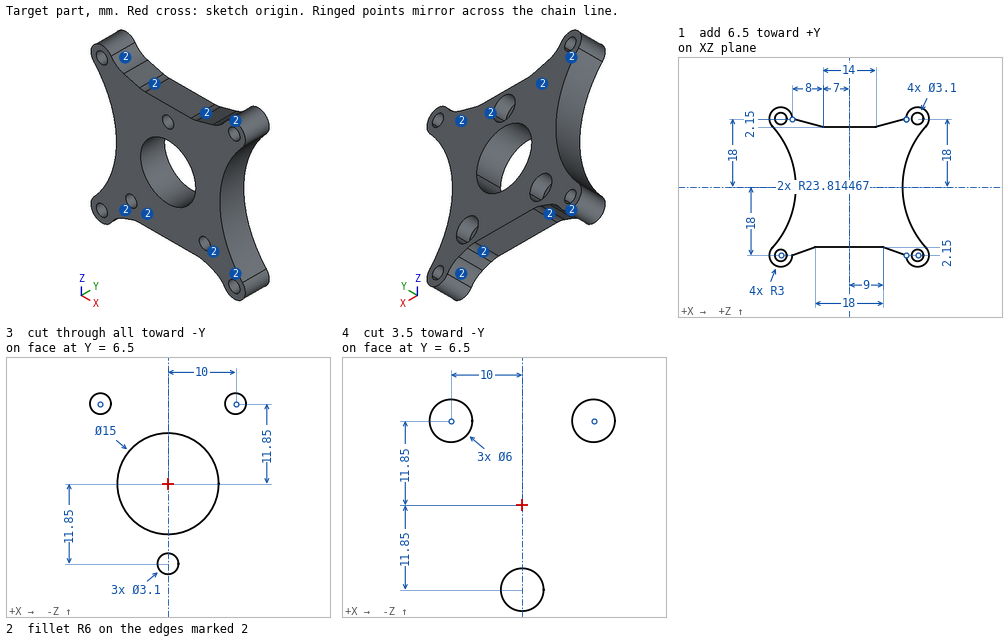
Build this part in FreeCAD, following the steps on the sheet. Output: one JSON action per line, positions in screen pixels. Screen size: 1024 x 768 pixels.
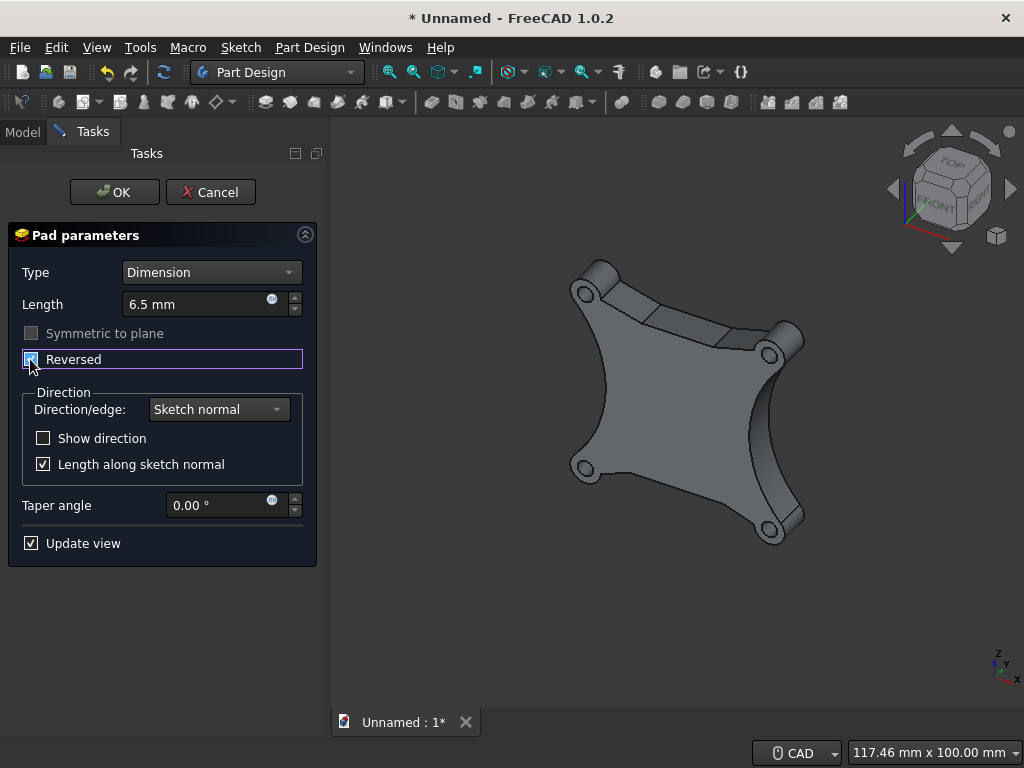
{"action": "left_click", "coordinate": [115, 192]}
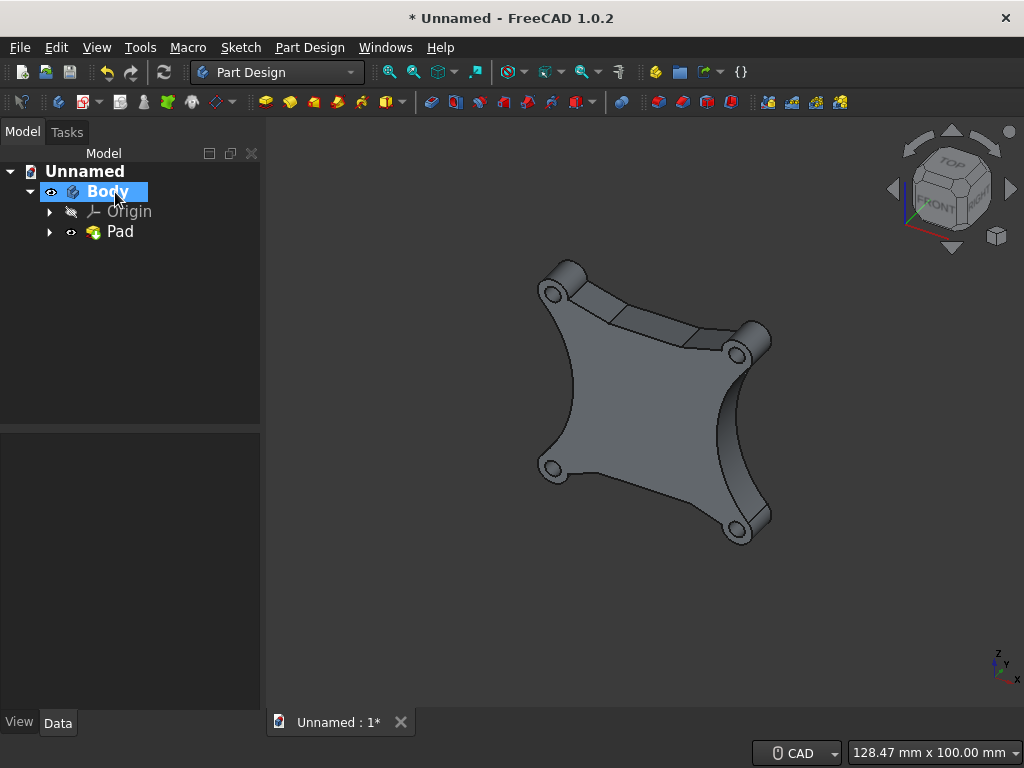
{"action": "key", "text": "0"}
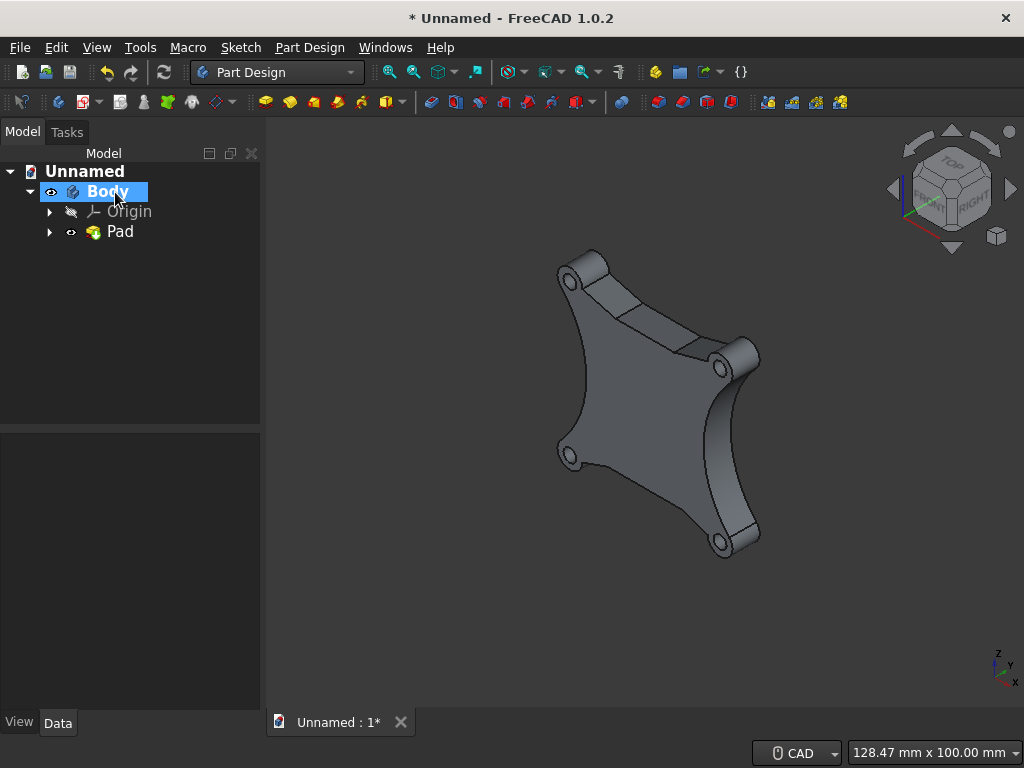
{"action": "key", "text": "2"}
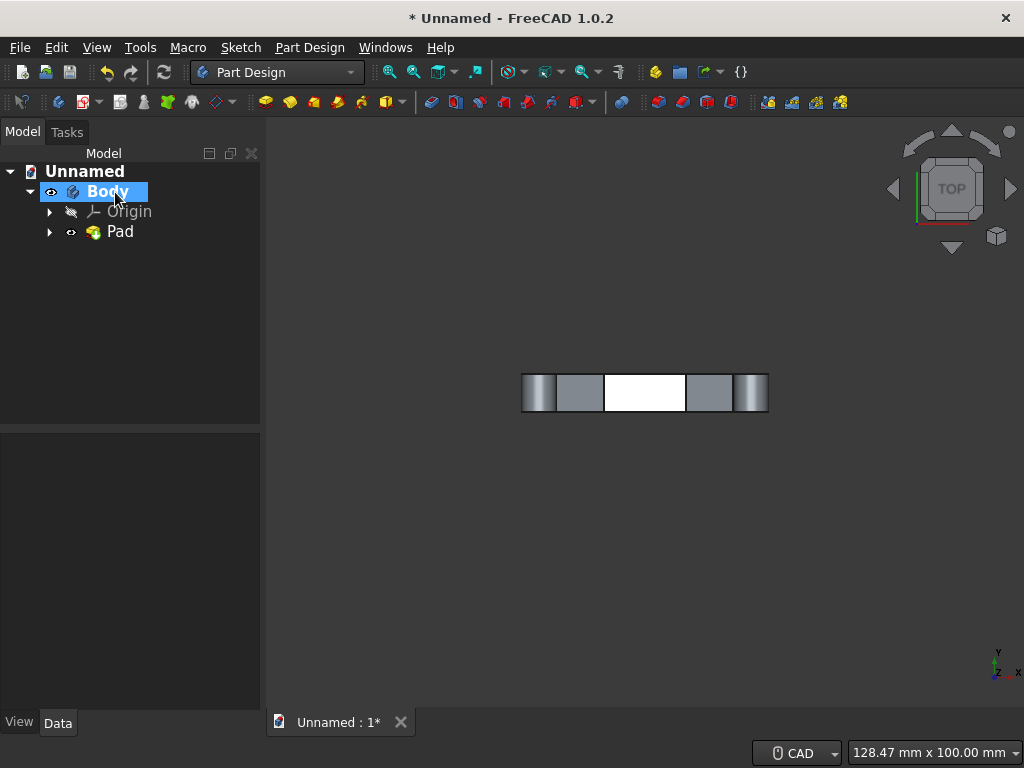
{"action": "left_click", "coordinate": [390, 72]}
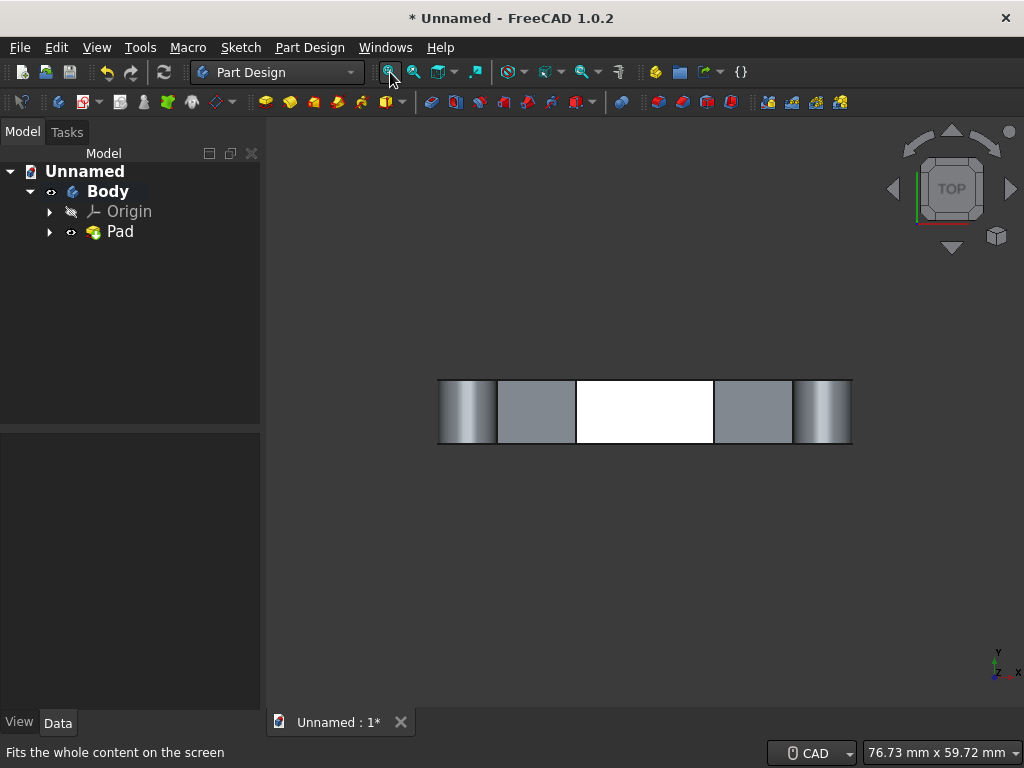
{"action": "key", "text": "1"}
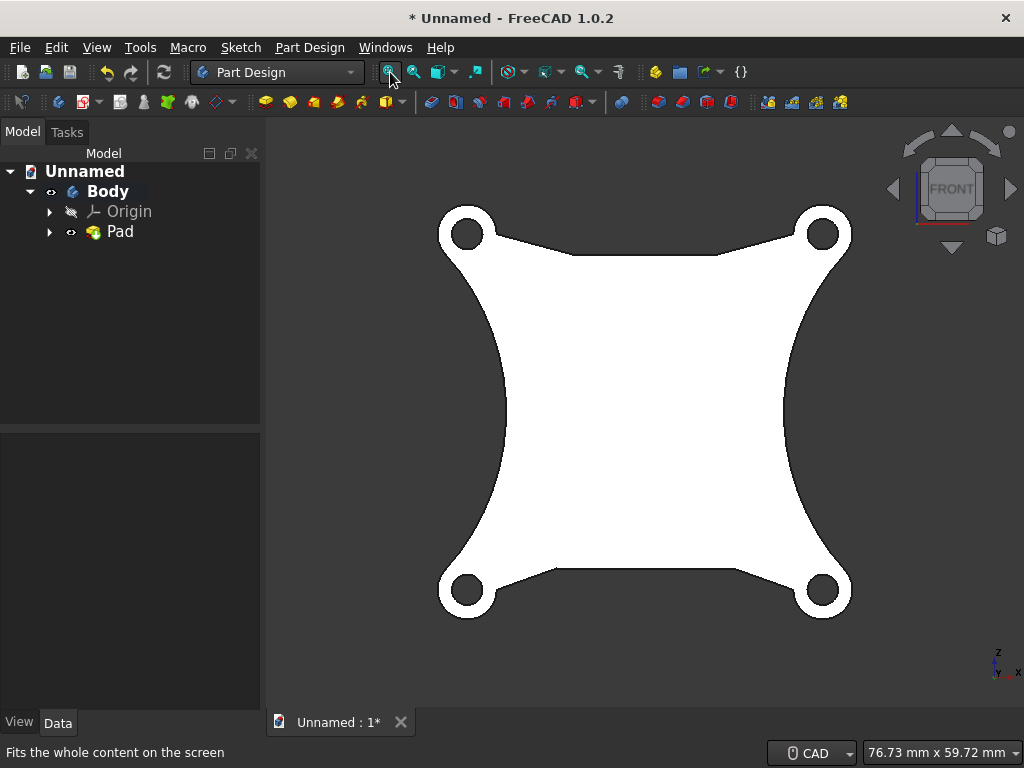
{"action": "key", "text": "3"}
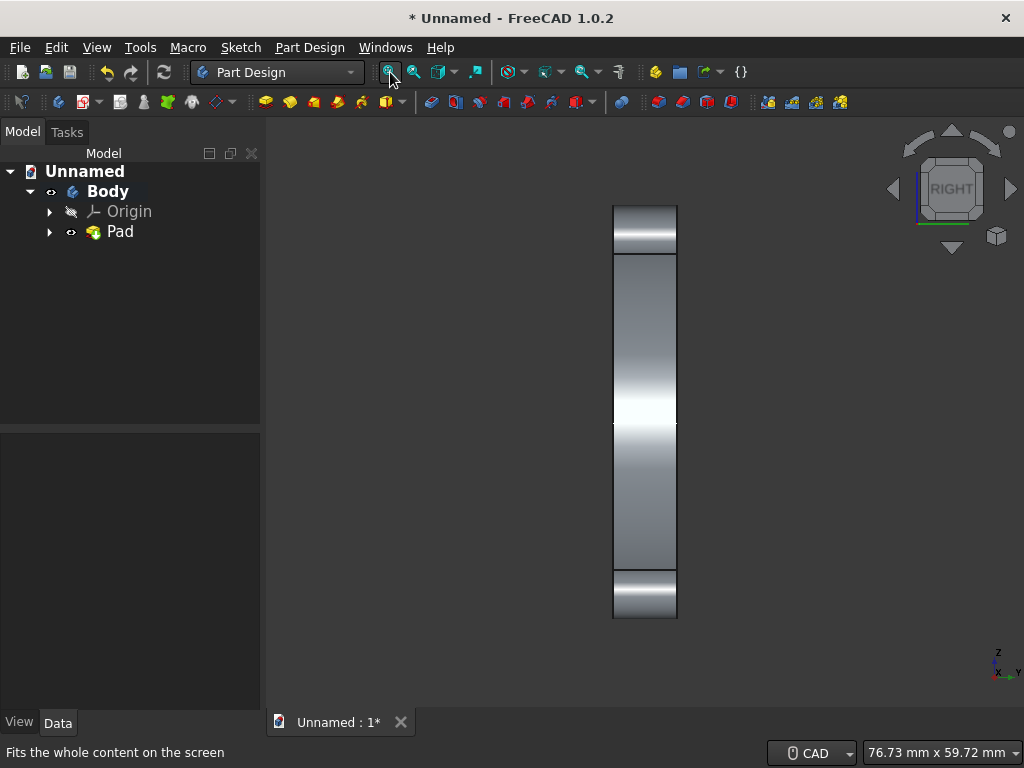
{"action": "key", "text": "5"}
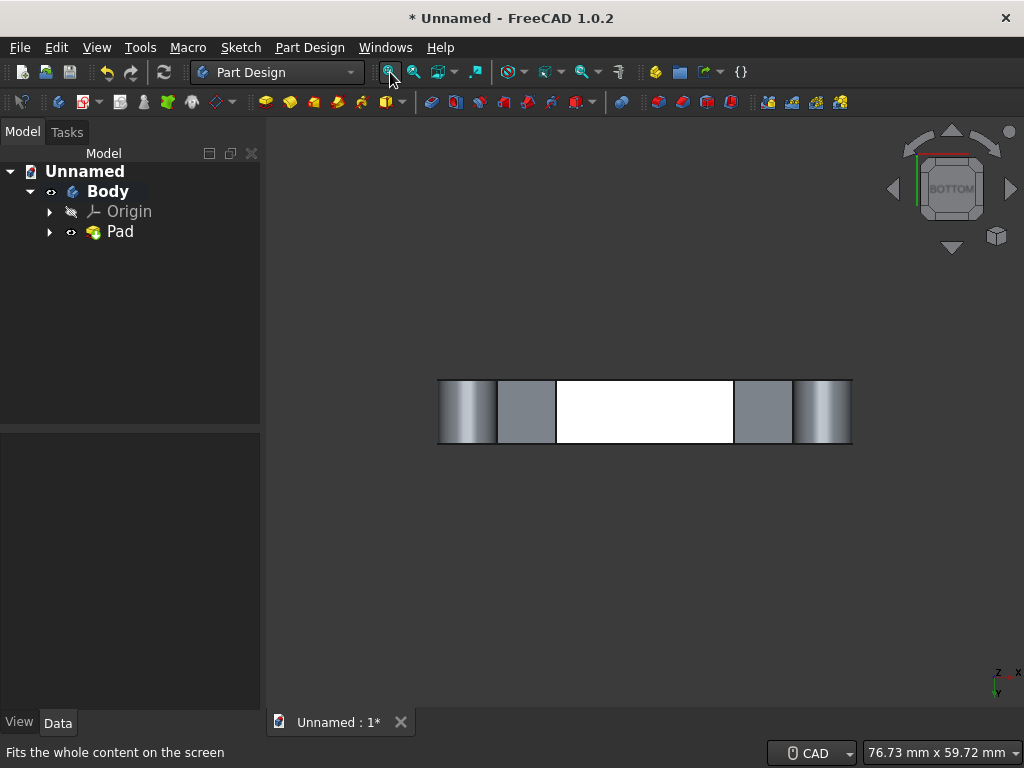
{"action": "key", "text": "4"}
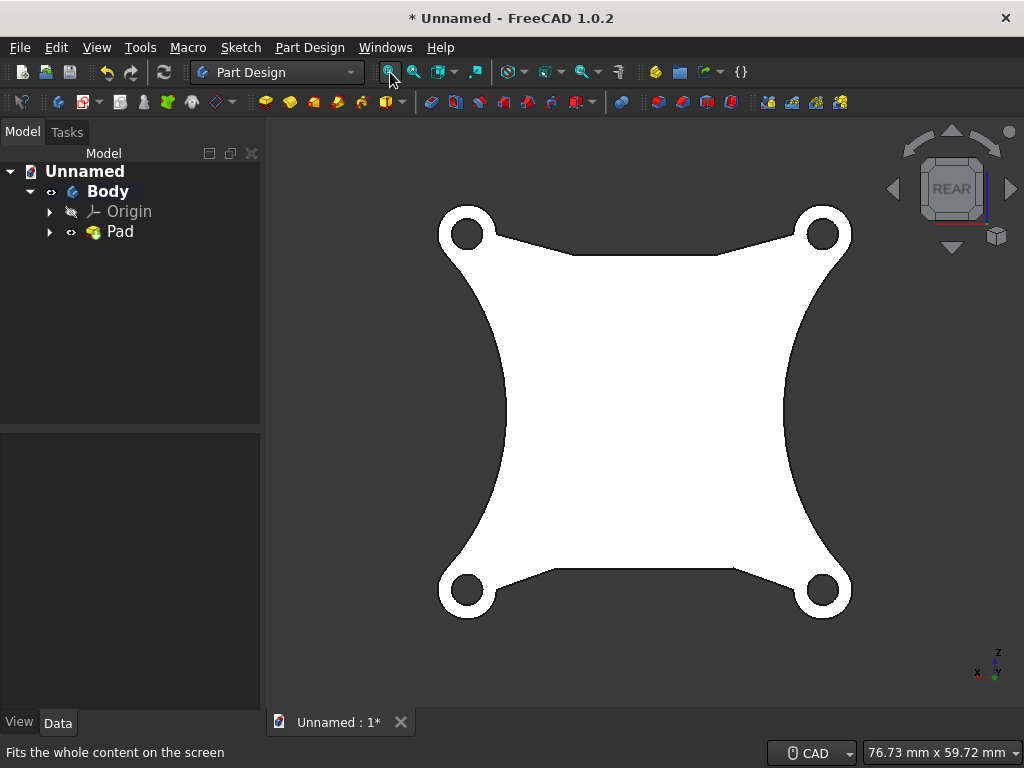
{"action": "key", "text": "6"}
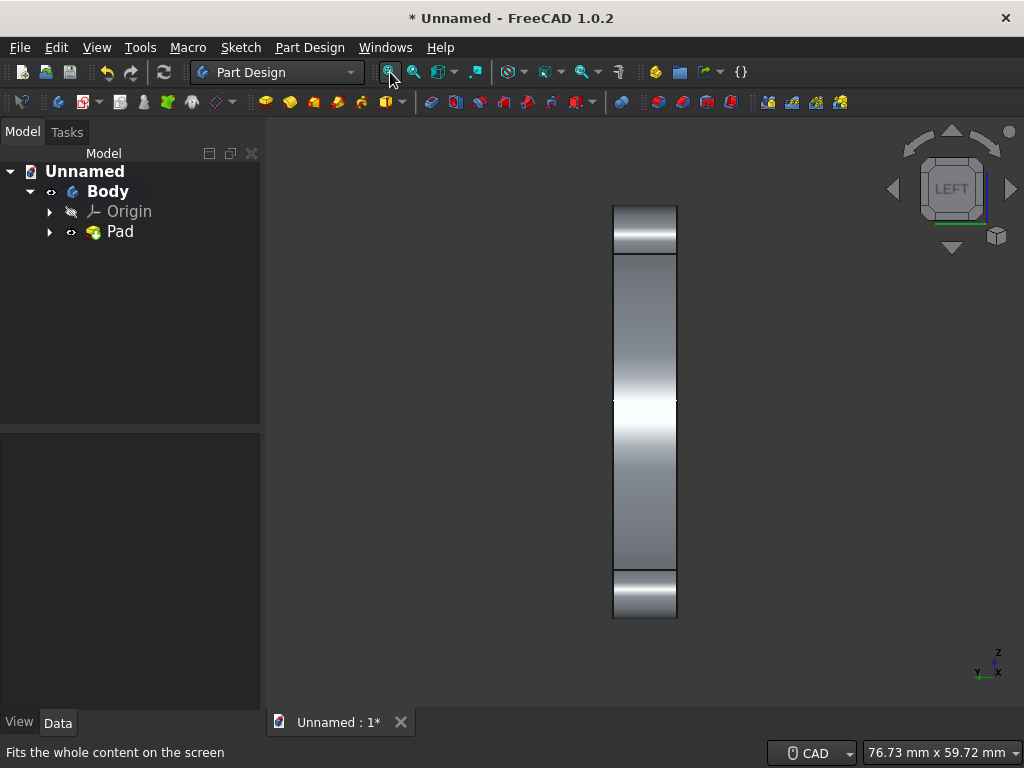
{"action": "key", "text": "v 3"}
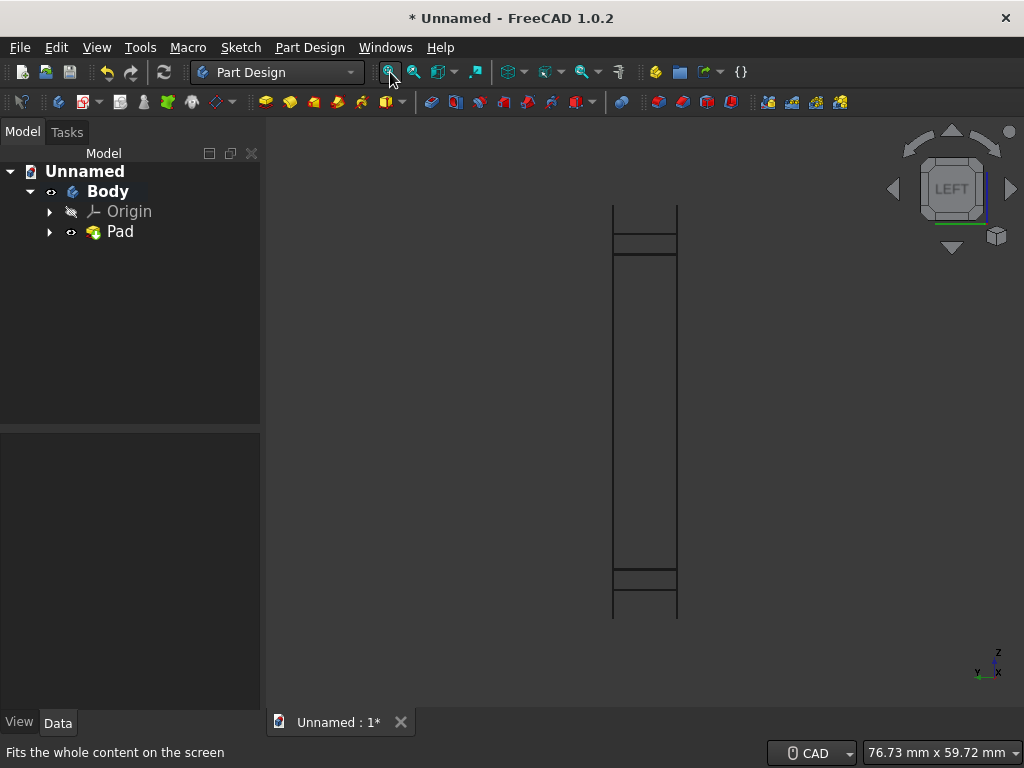
{"action": "key", "text": "0"}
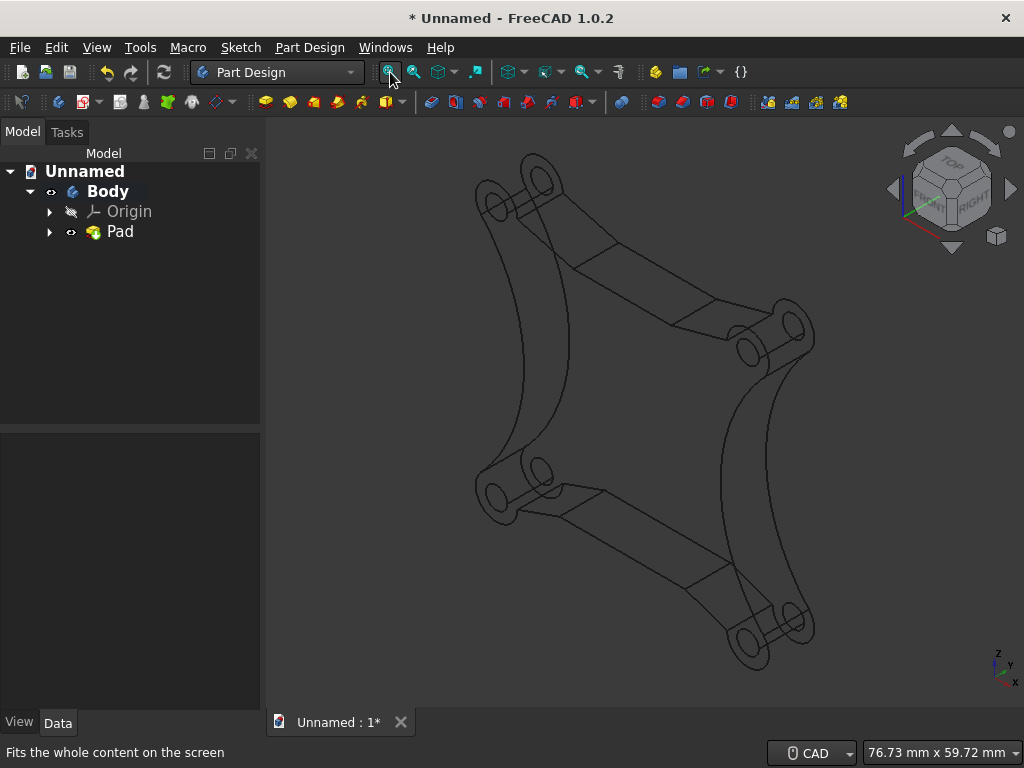
{"action": "left_click", "coordinate": [759, 321]}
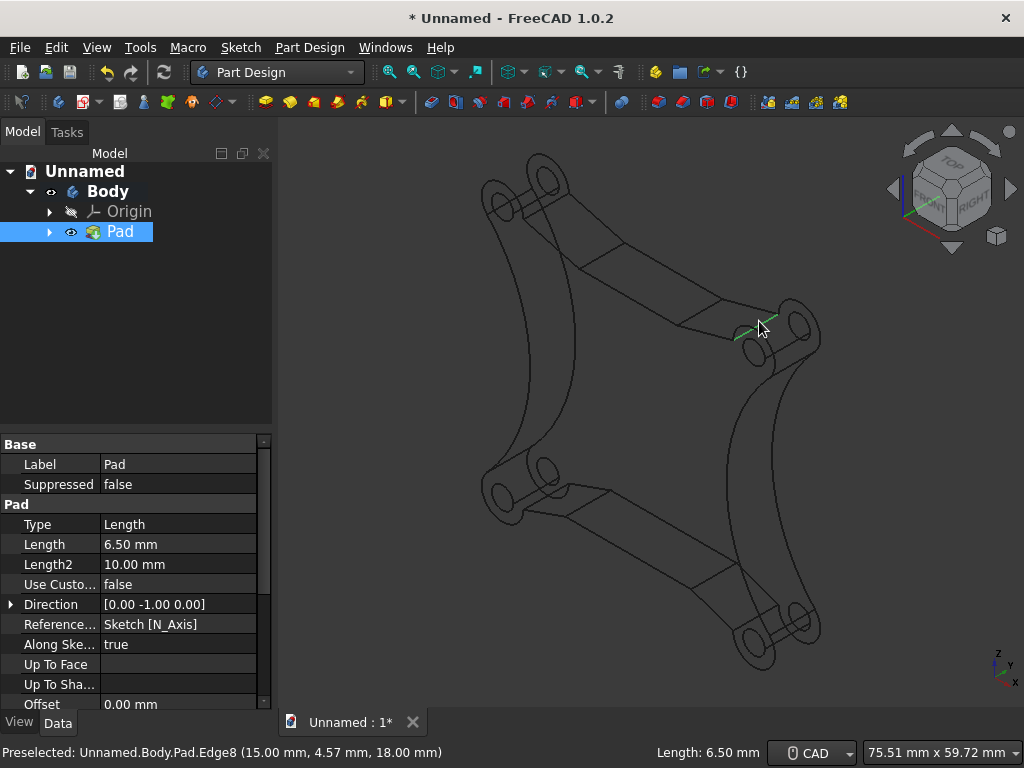
{"action": "left_click", "coordinate": [700, 311], "text": "ctrl"}